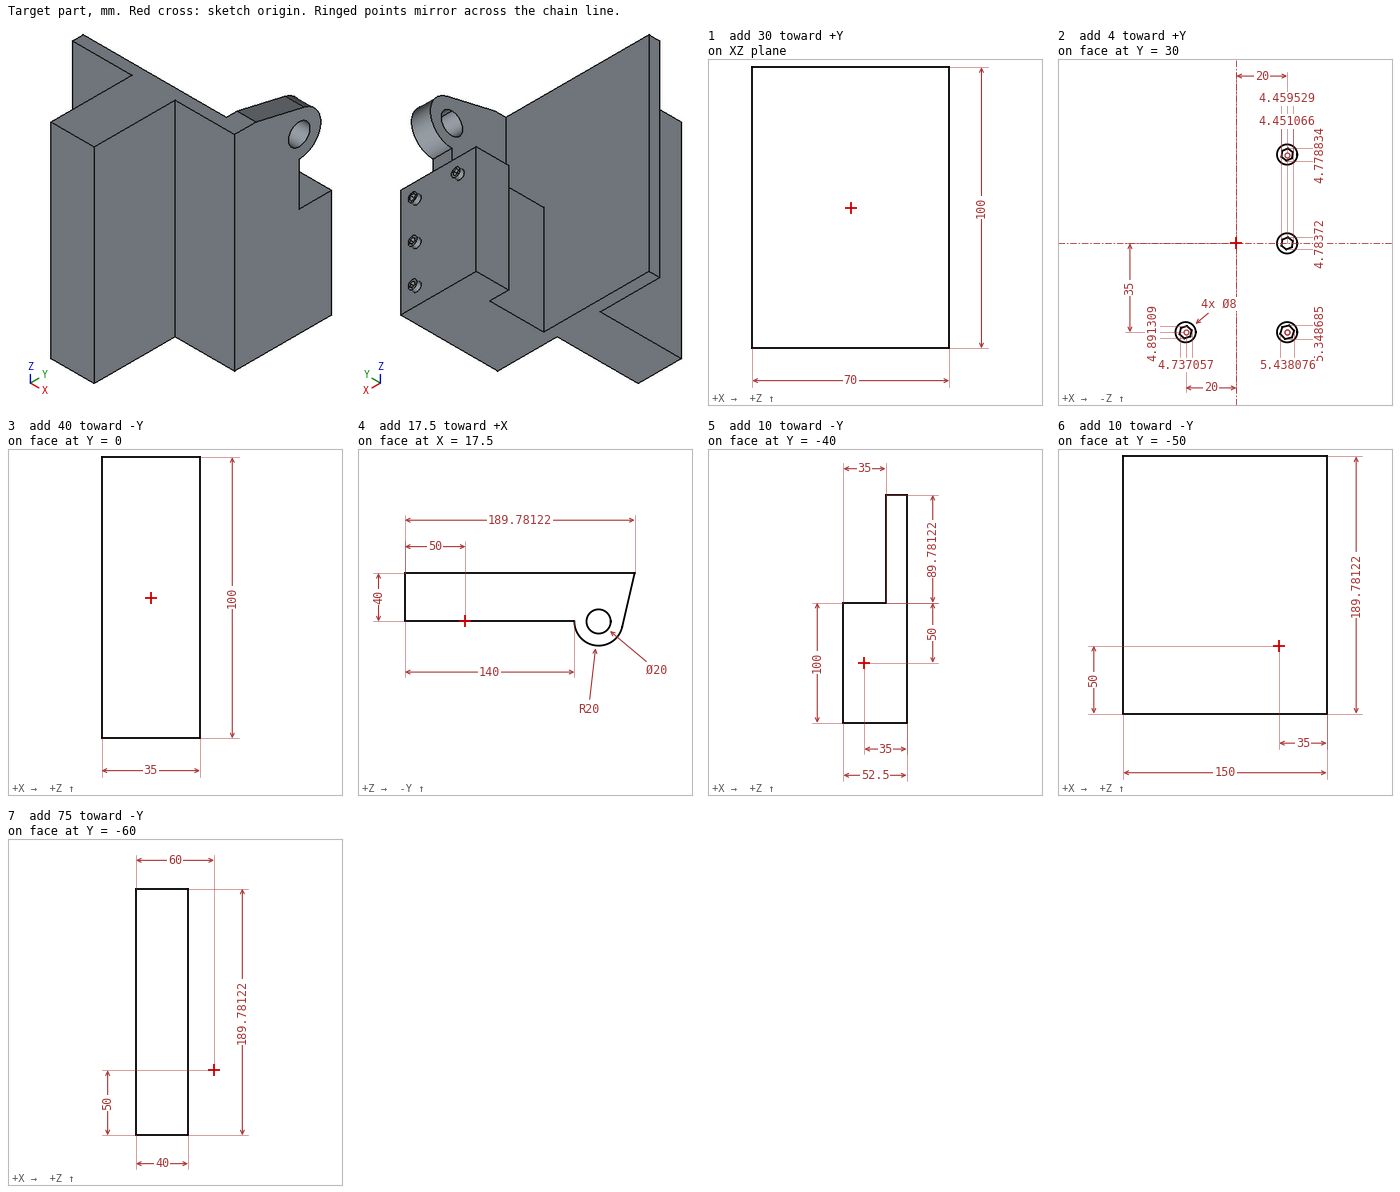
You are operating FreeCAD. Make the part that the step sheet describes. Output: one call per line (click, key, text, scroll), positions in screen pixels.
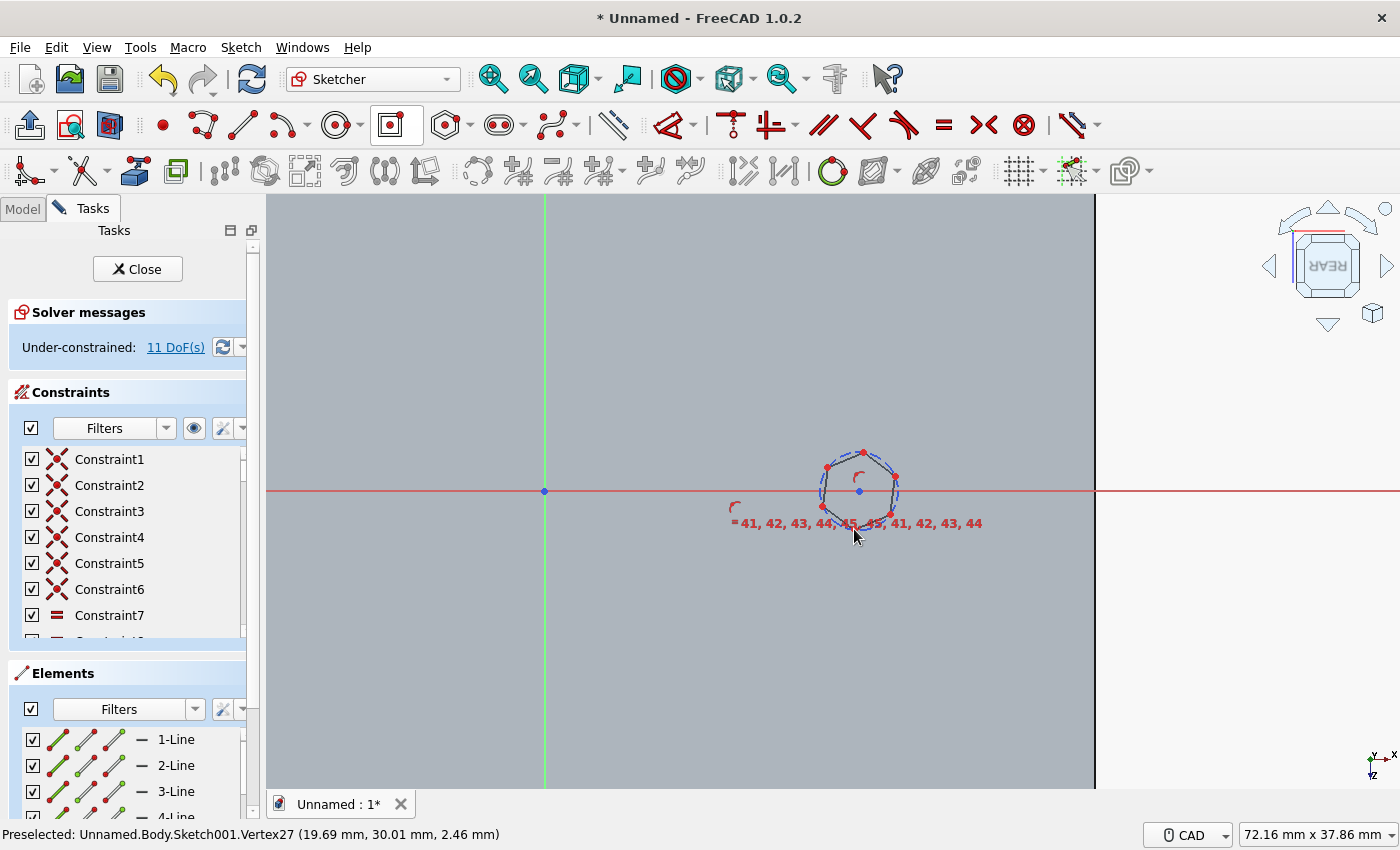
key(g)
key(p)
key(6)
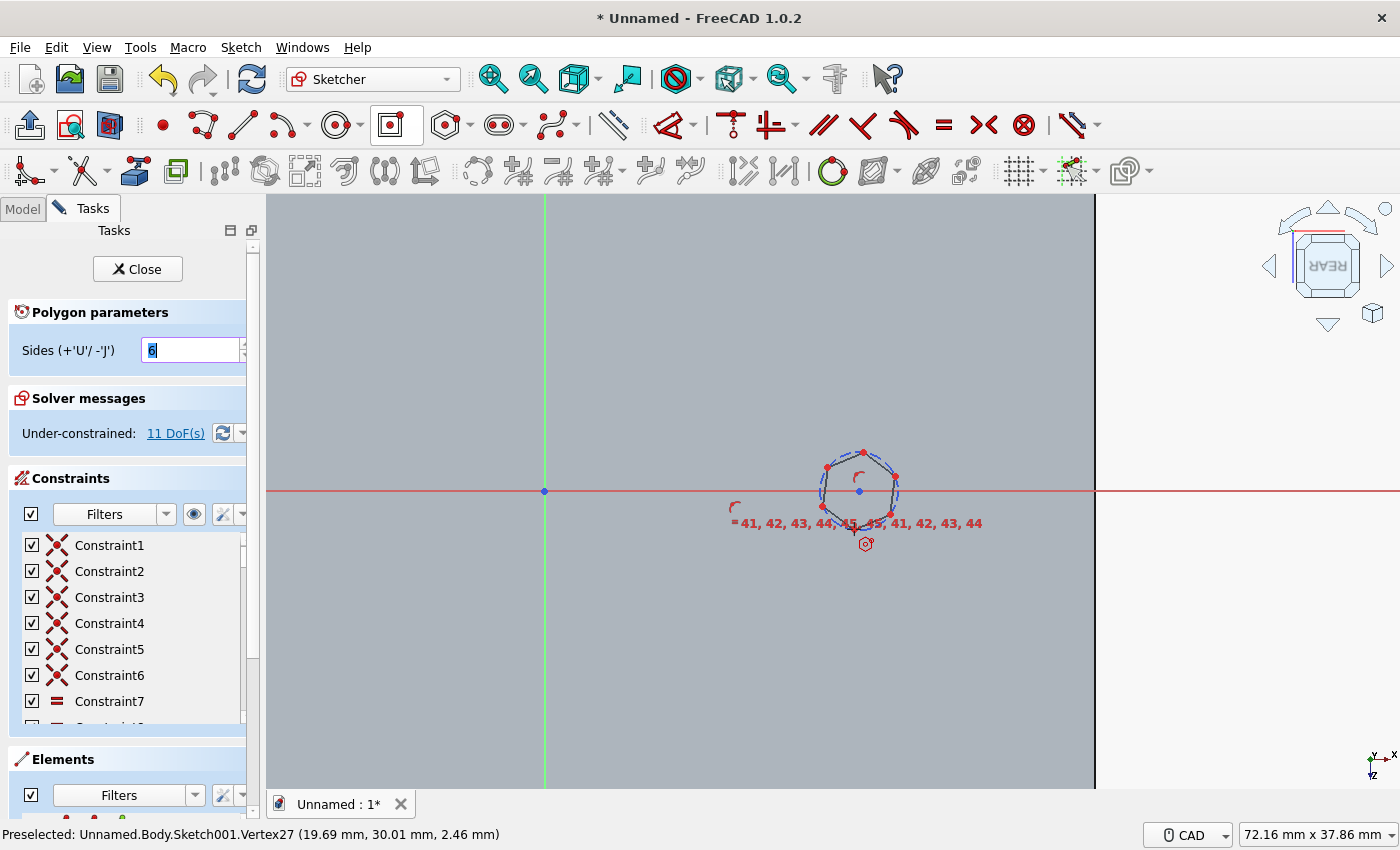
scroll(859, 492, down, 6)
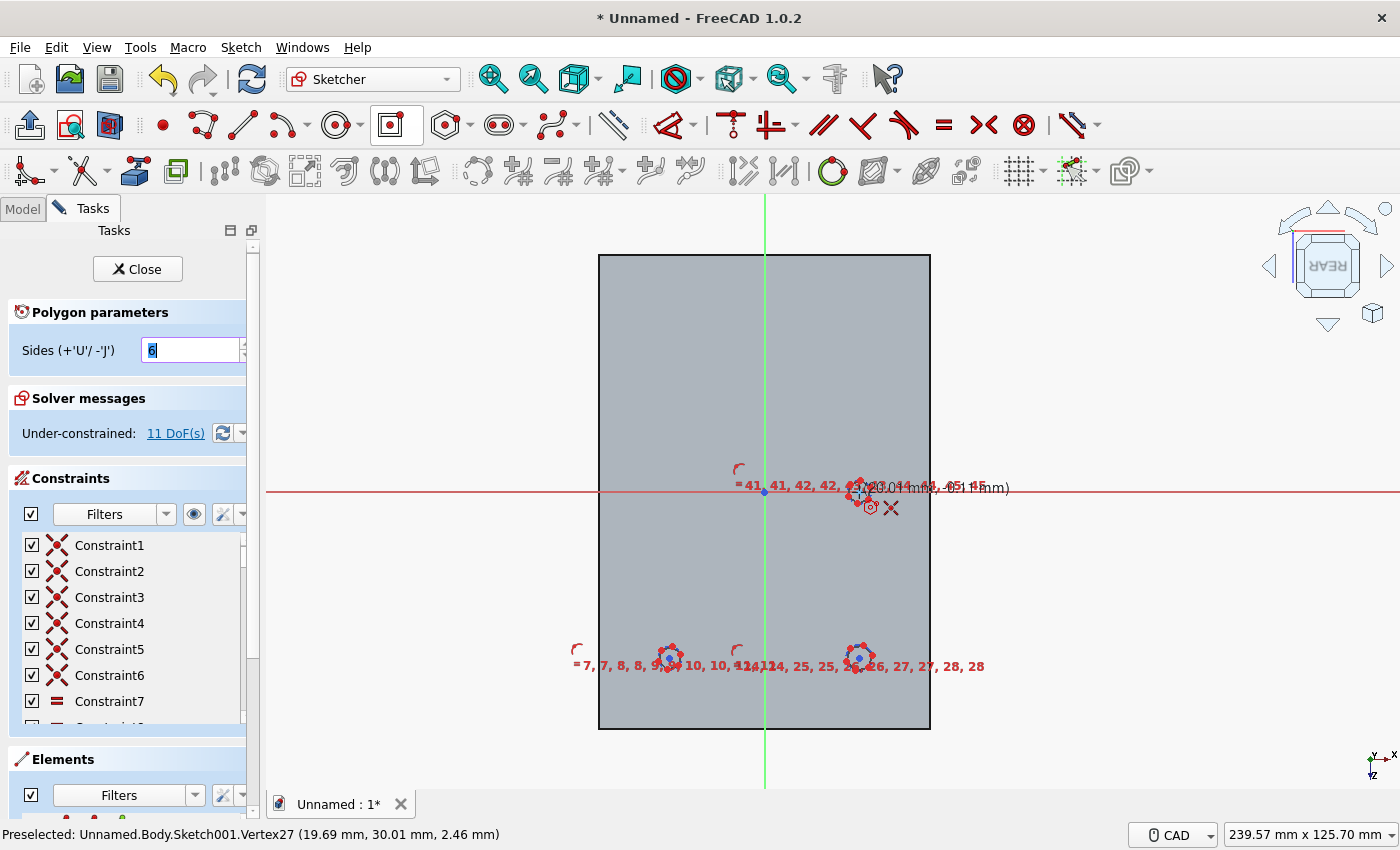
scroll(859, 326, up, 6)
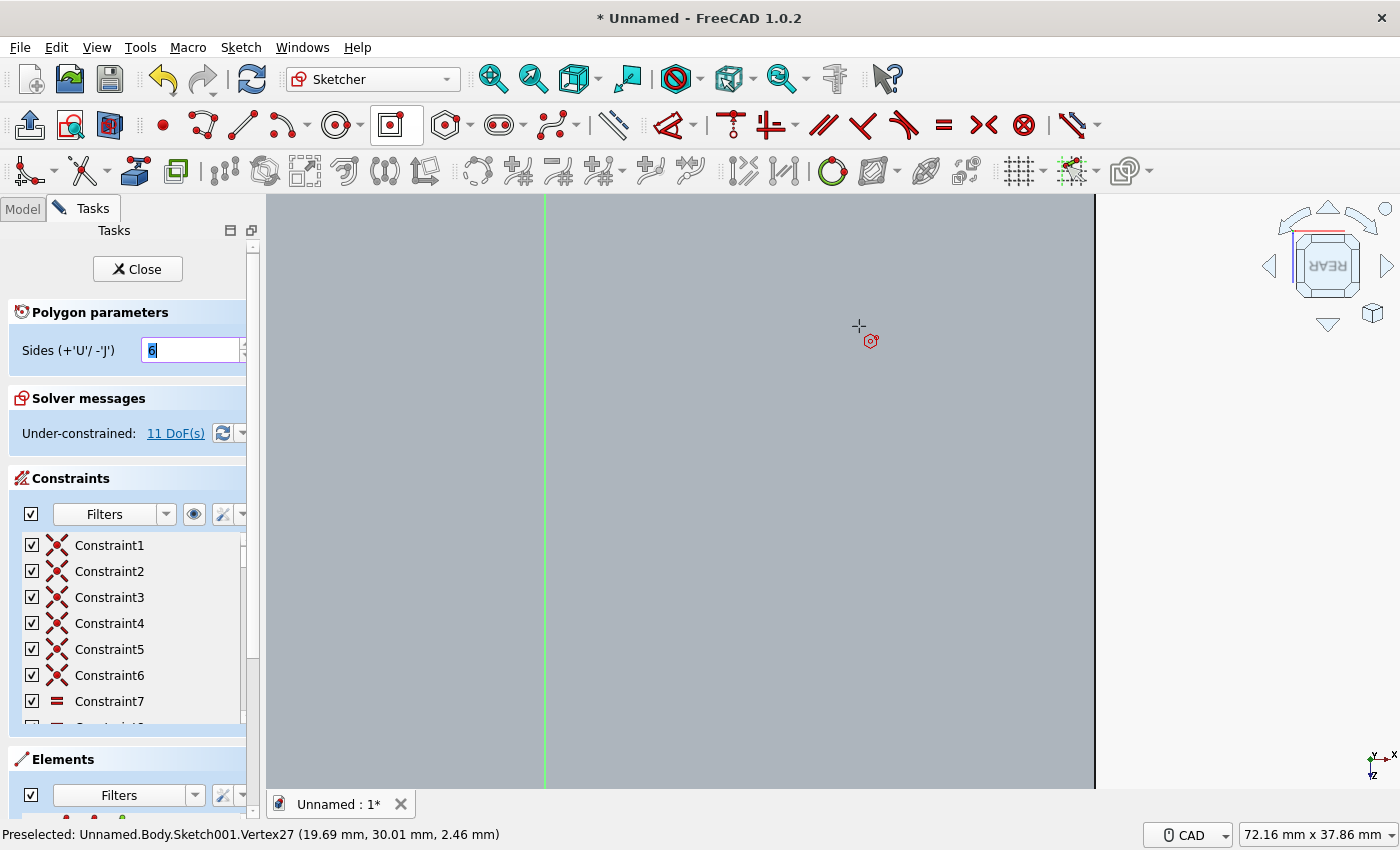
click(859, 327)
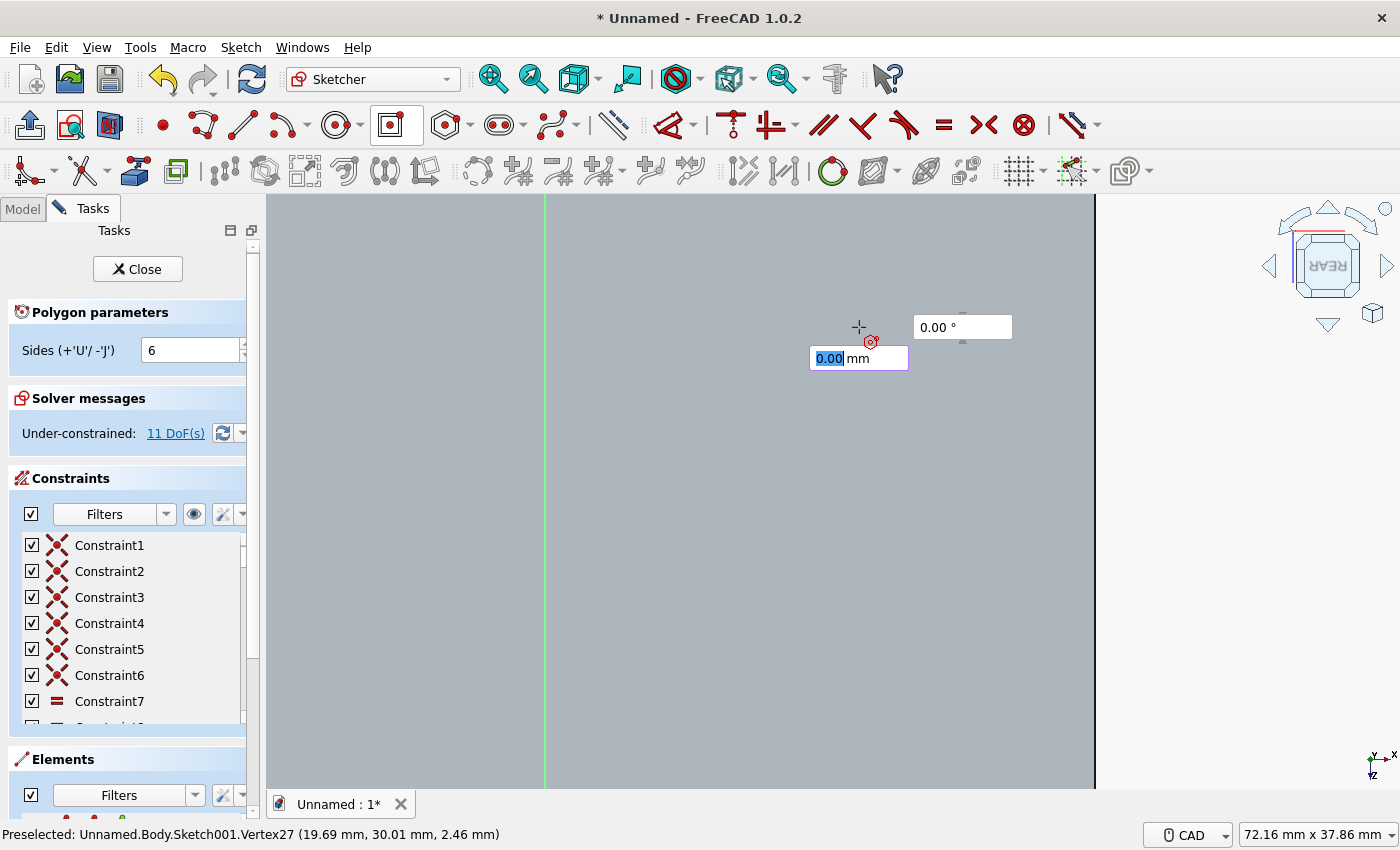
click(894, 312)
right_click(894, 312)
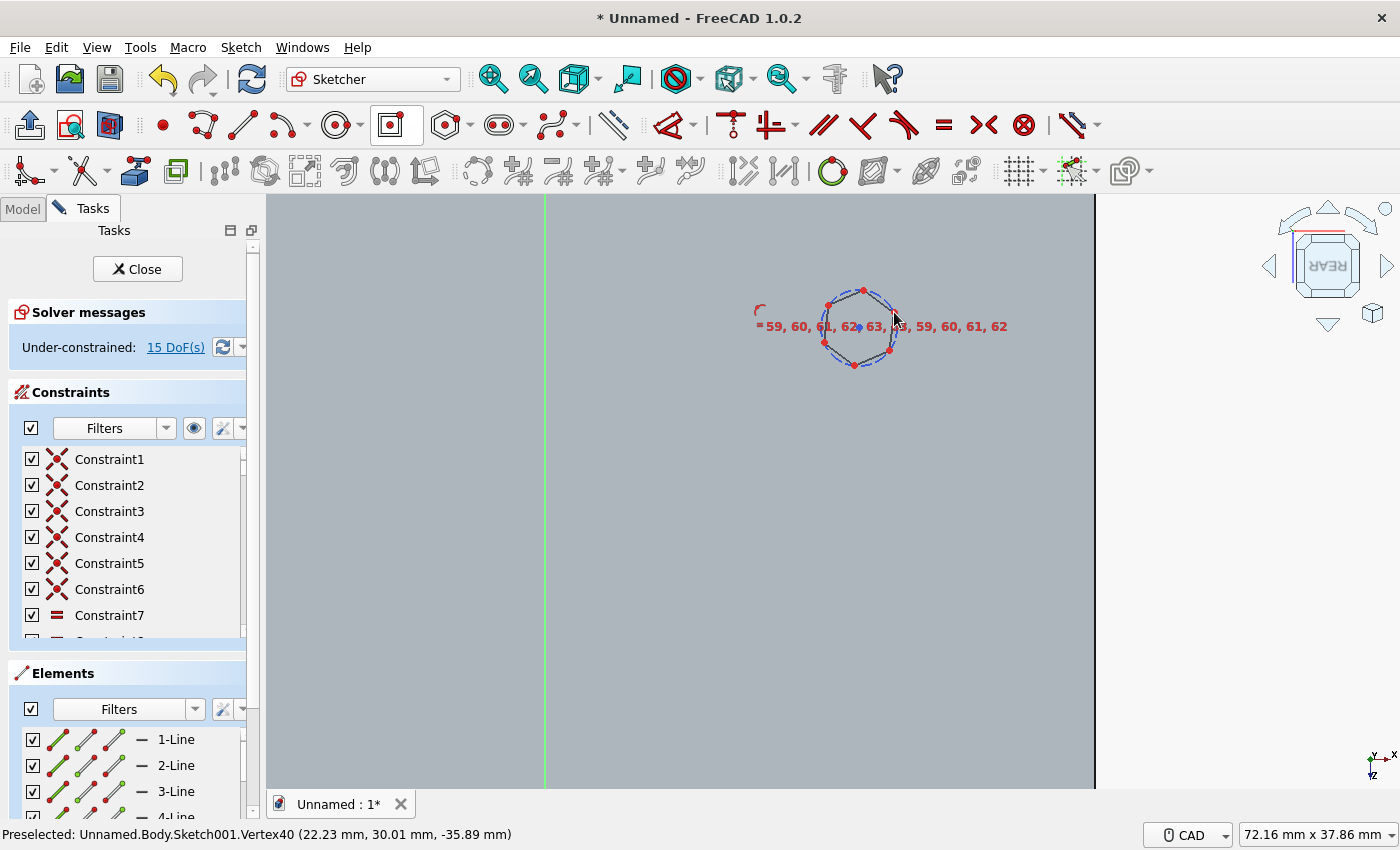
click(336, 126)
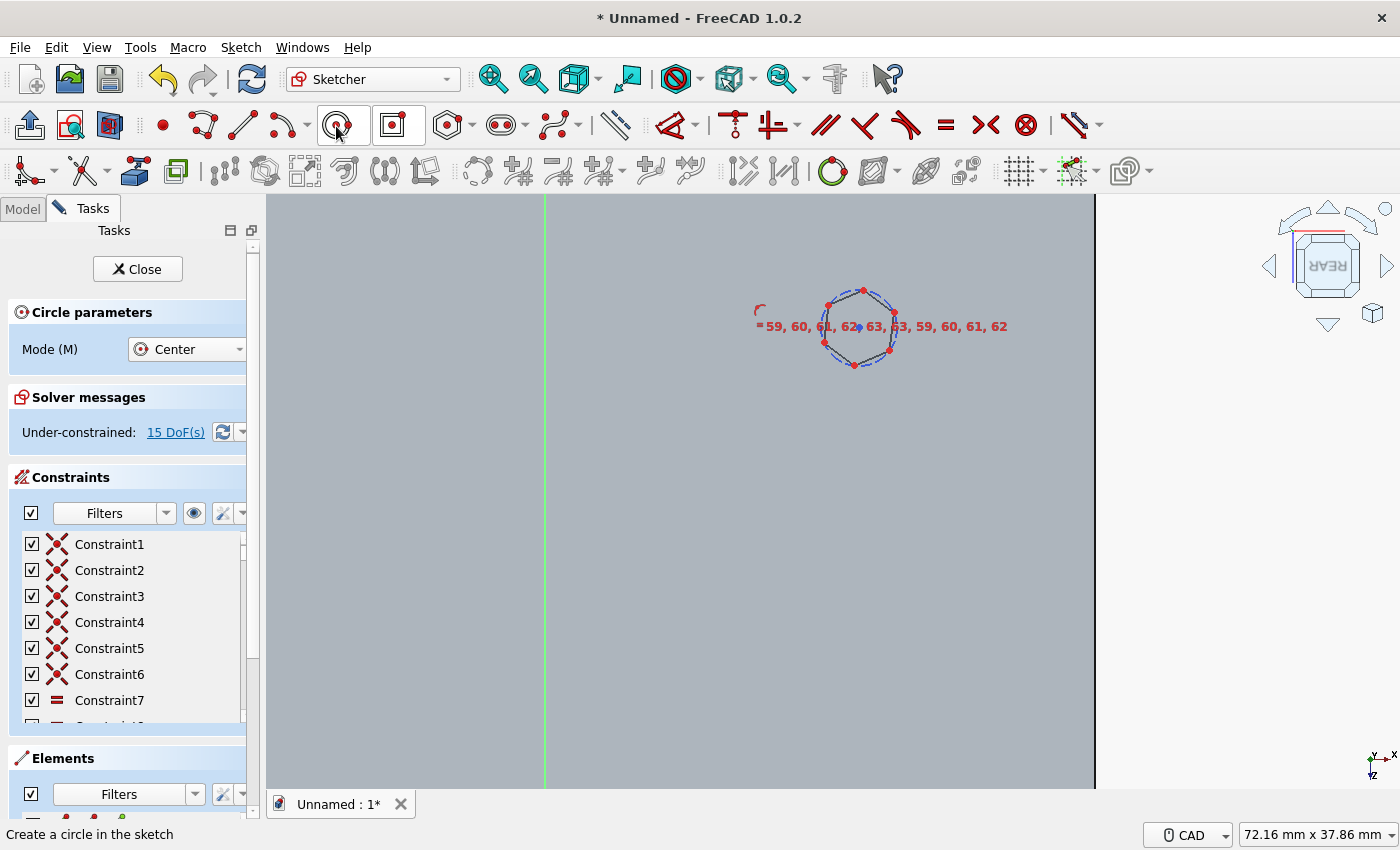
scroll(859, 325, down, 6)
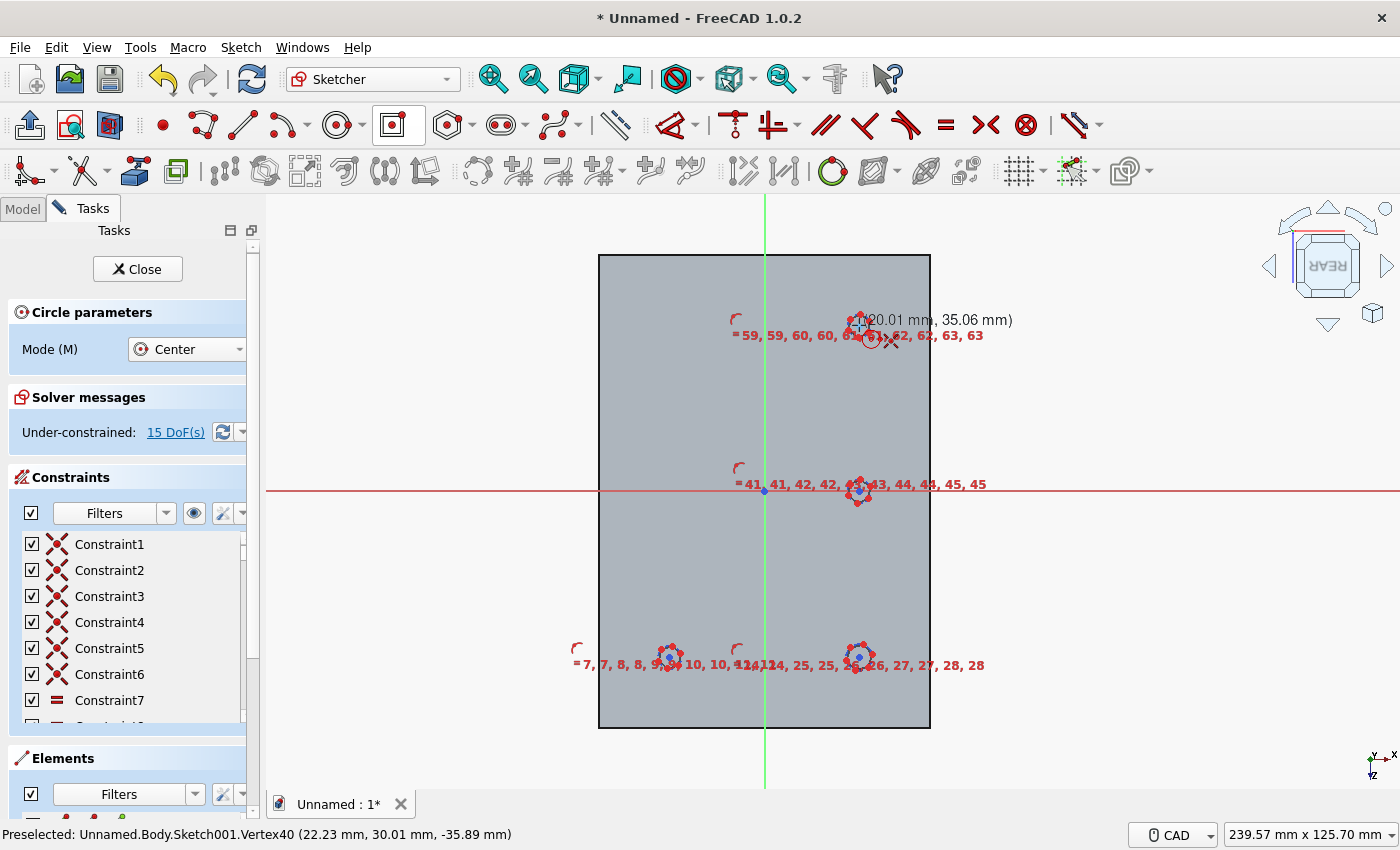
scroll(670, 657, up, 3)